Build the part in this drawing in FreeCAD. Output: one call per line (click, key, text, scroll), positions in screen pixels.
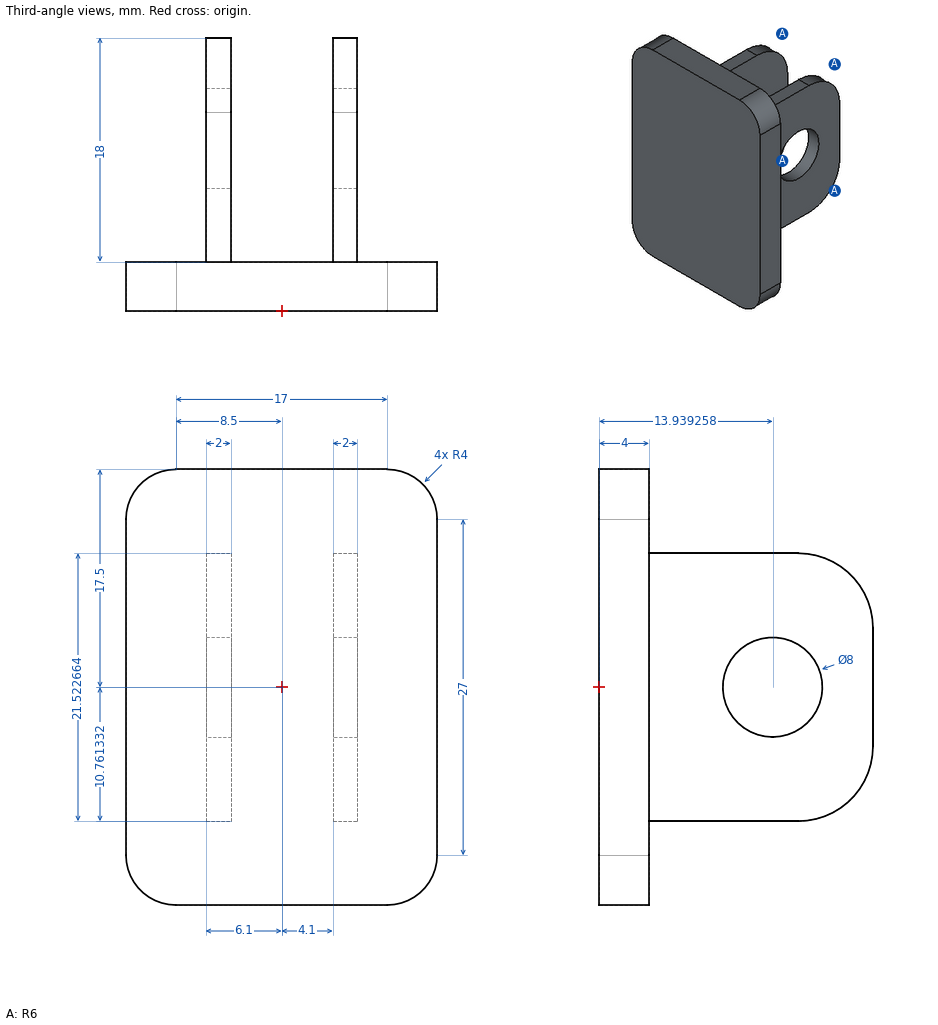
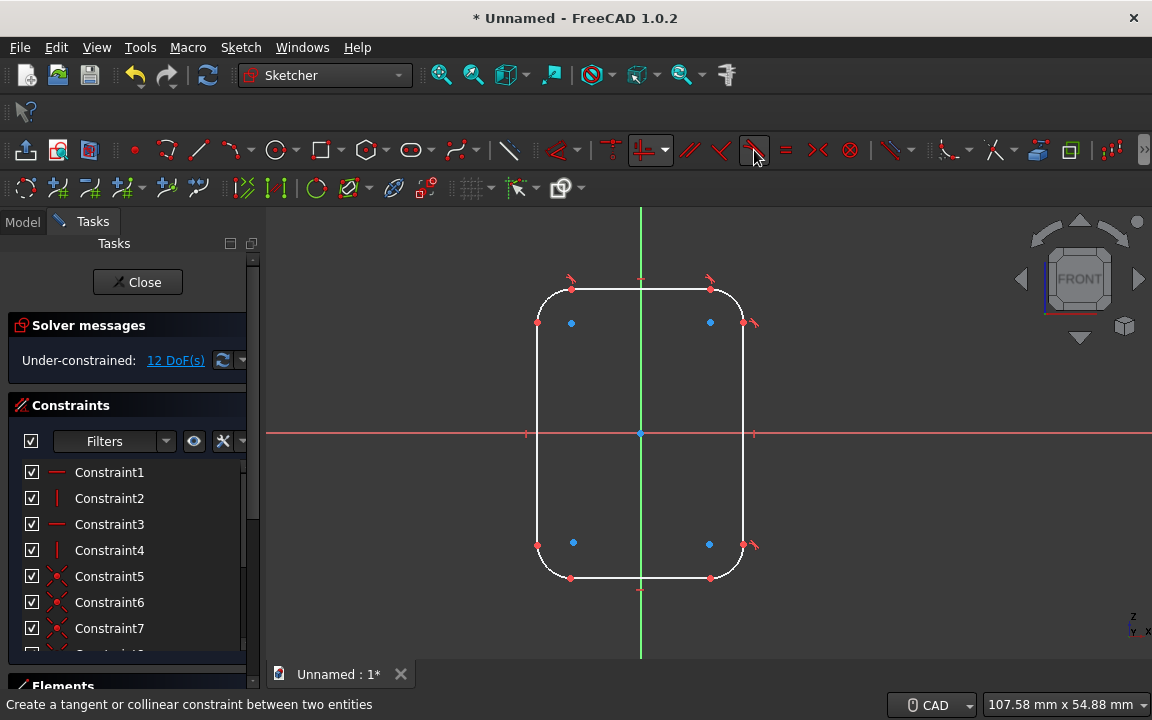
click(668, 578)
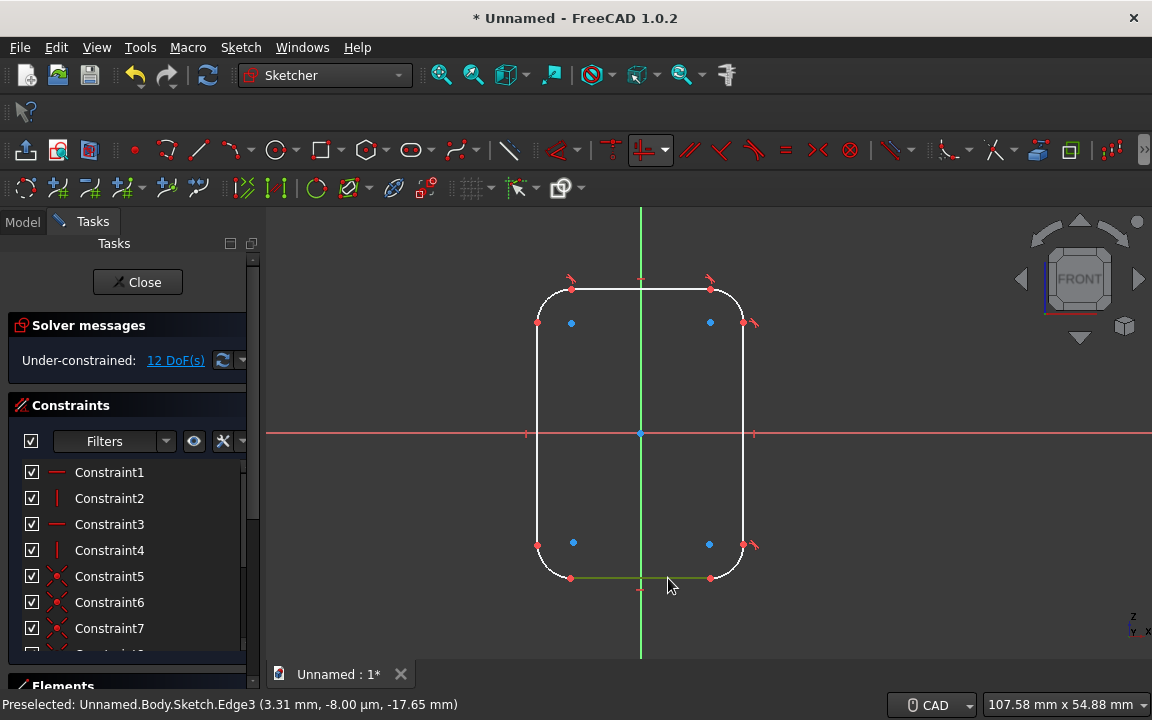
click(725, 574)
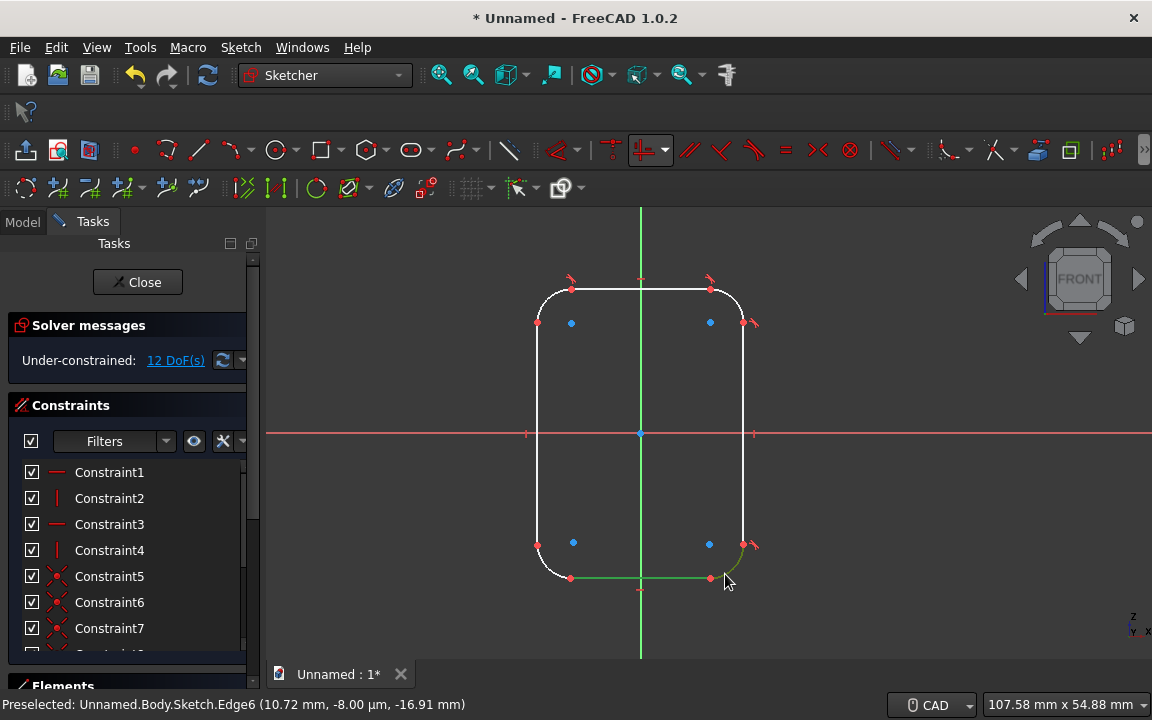
click(754, 150)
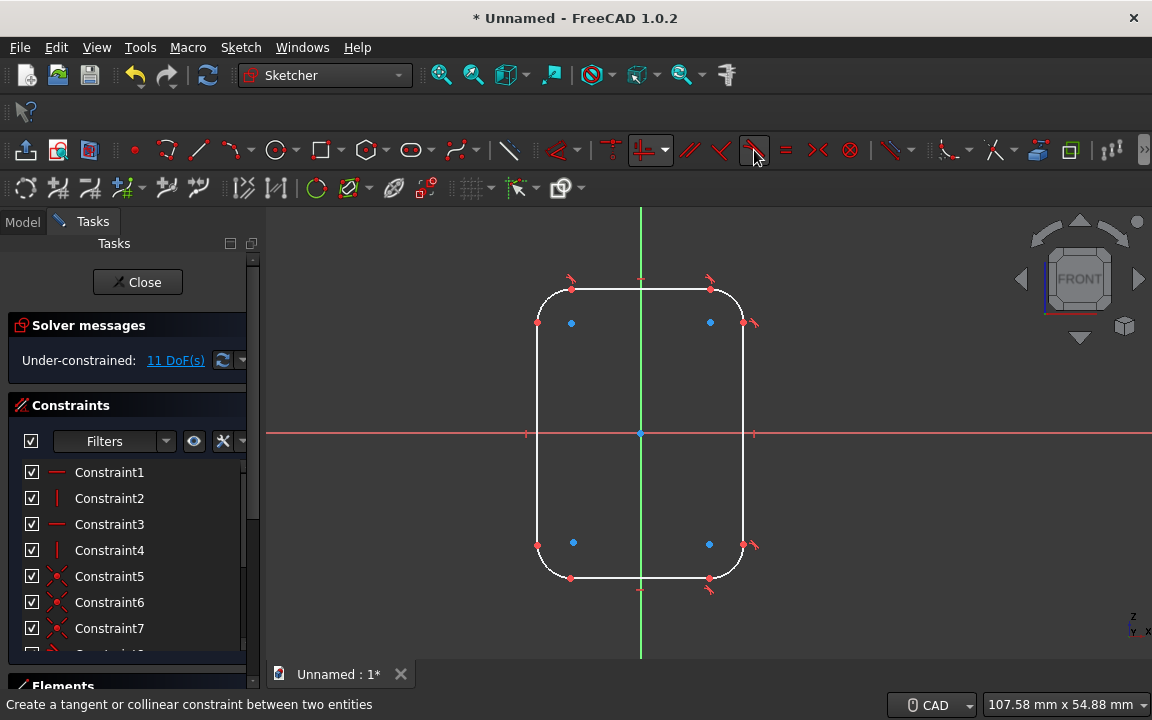
click(668, 578)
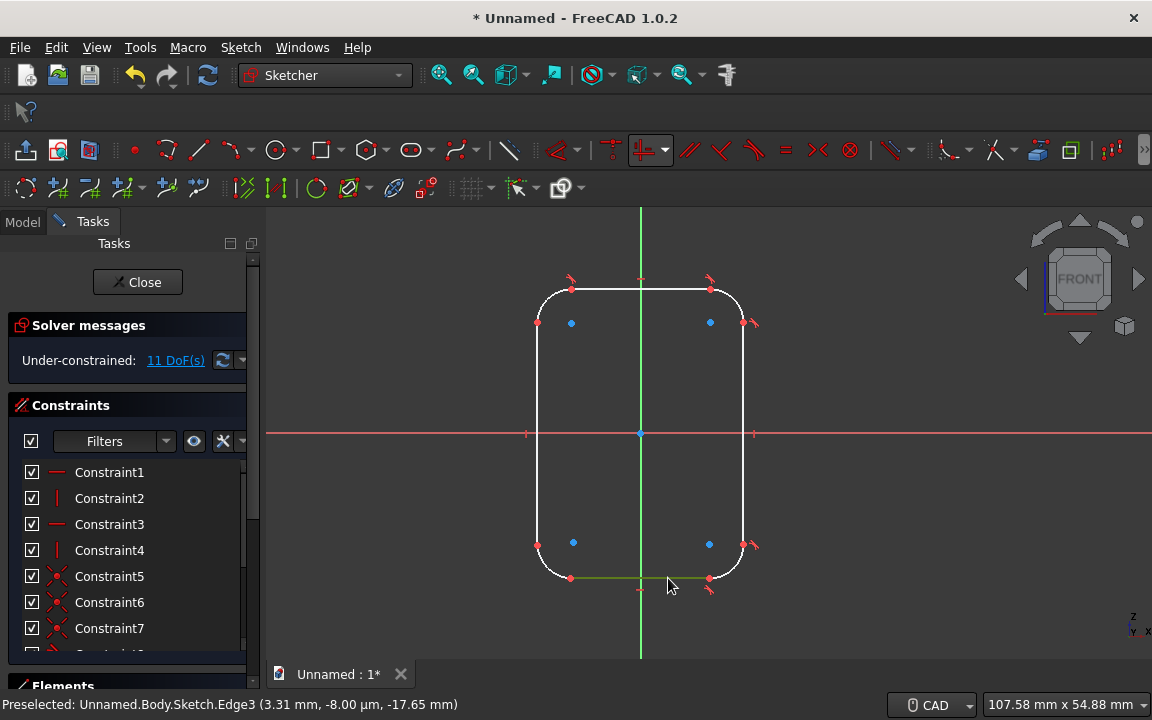
click(542, 560)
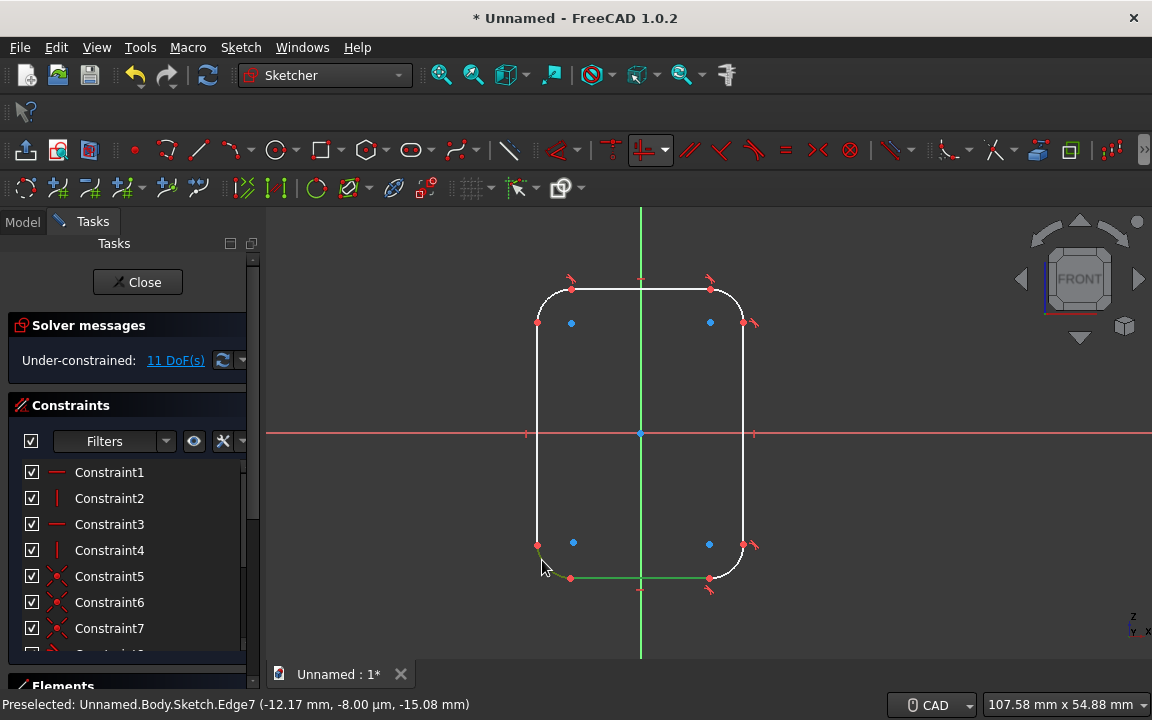
click(754, 150)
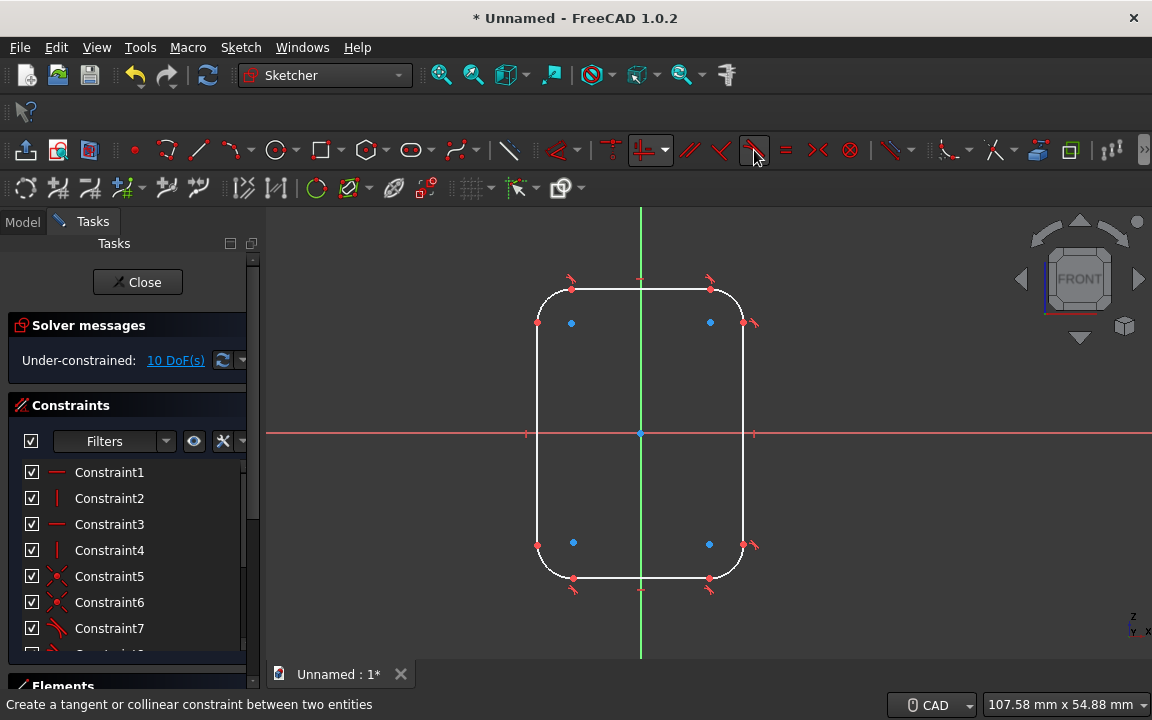
click(537, 479)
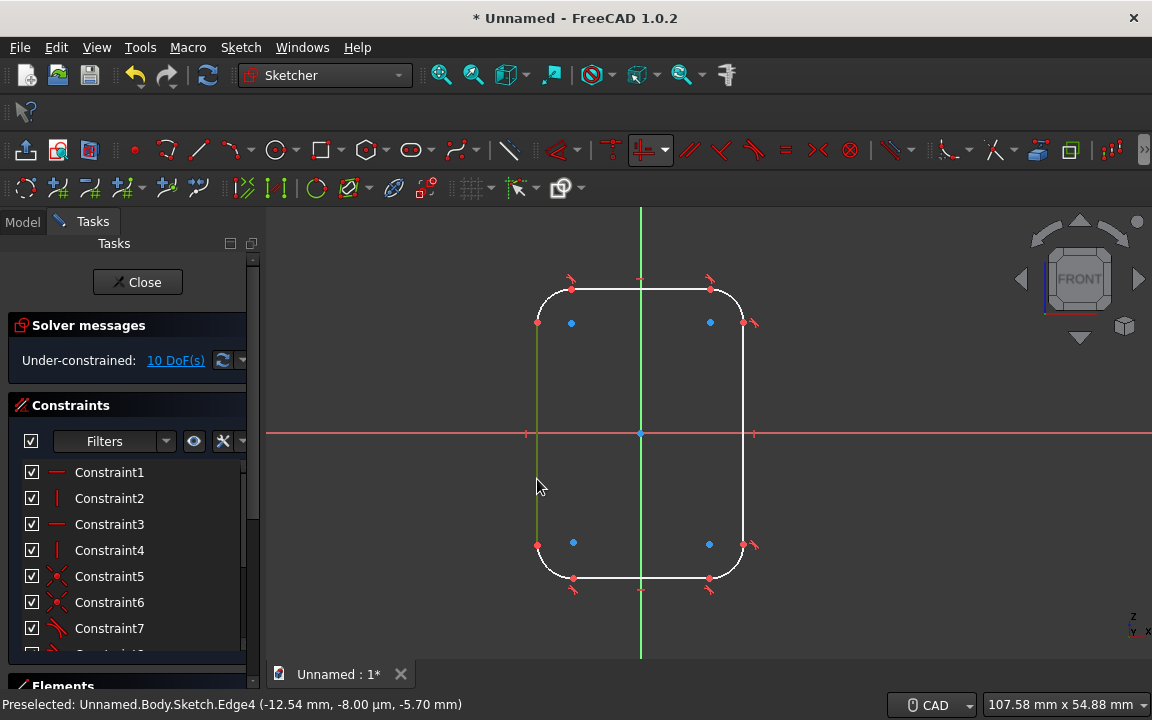
click(542, 561)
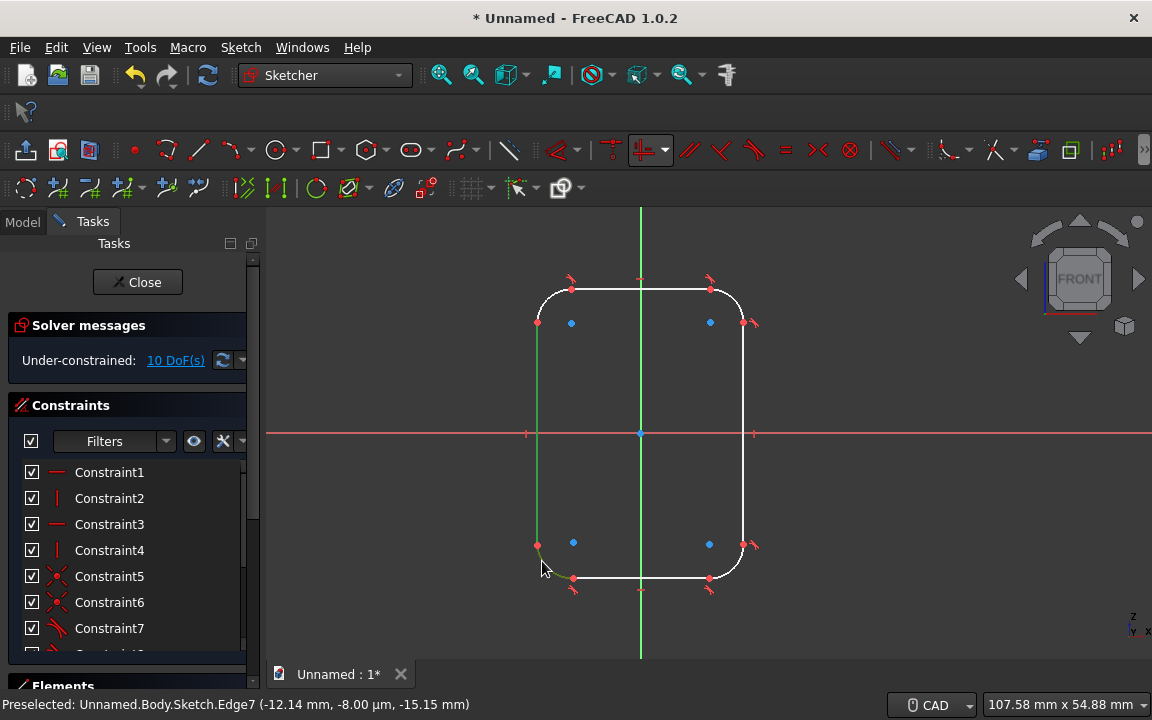
click(754, 150)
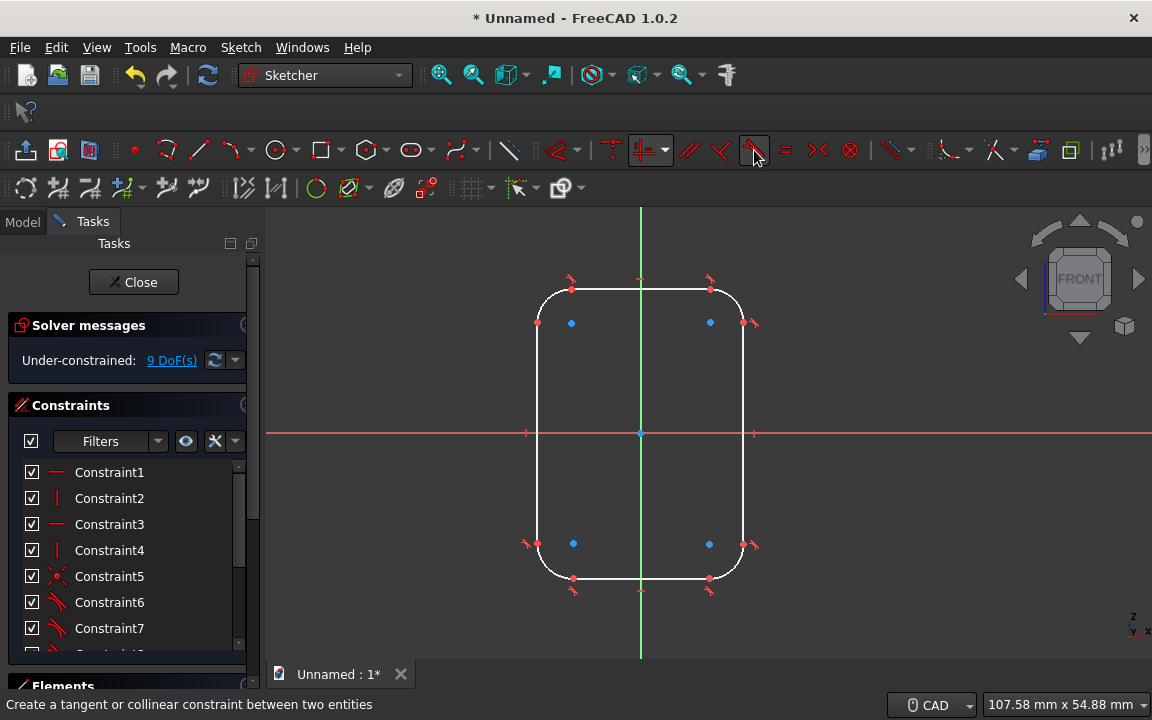
click(537, 477)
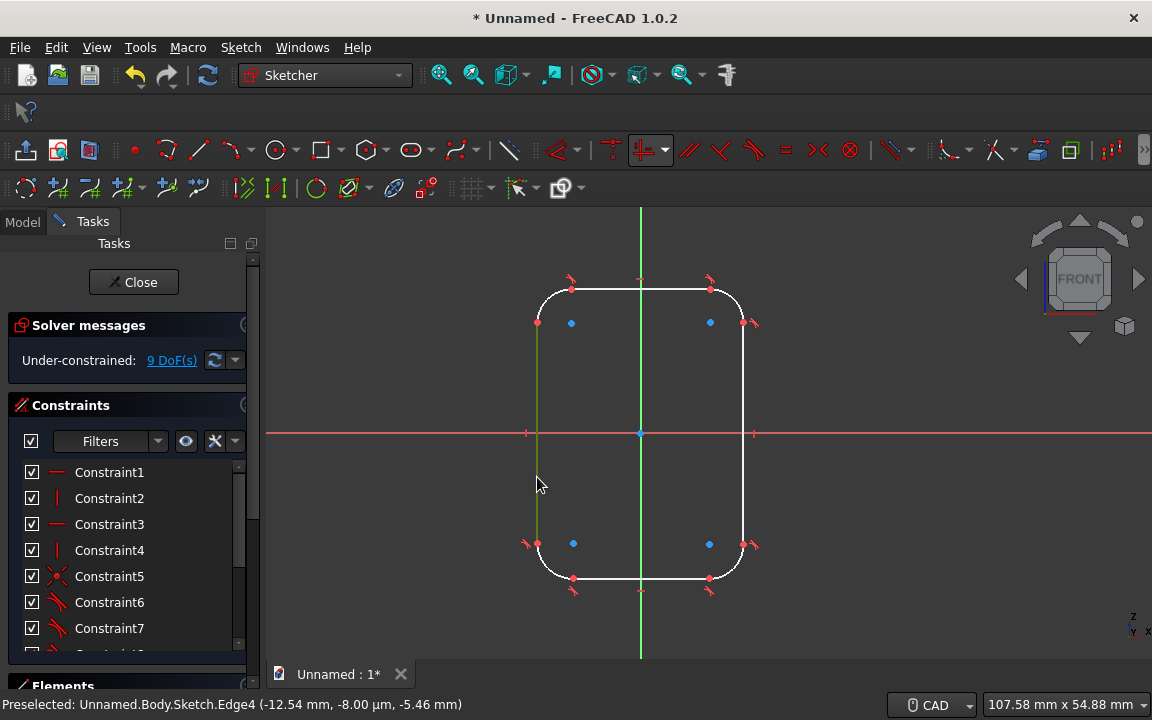
click(556, 293)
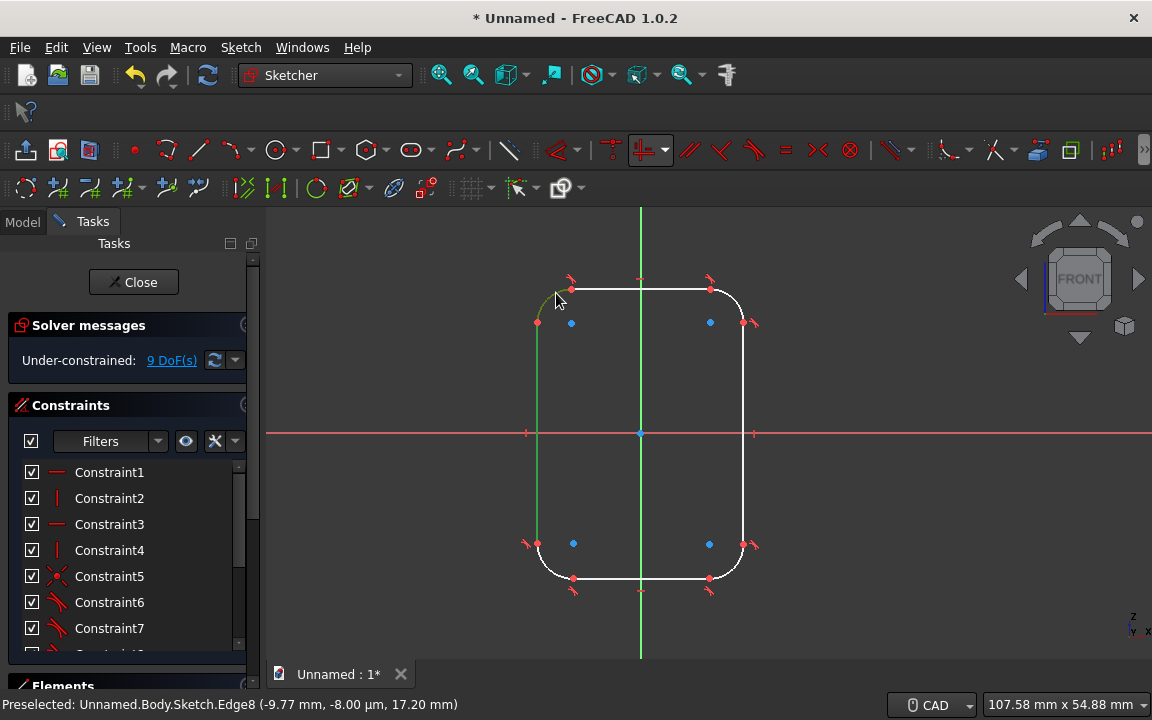
click(754, 150)